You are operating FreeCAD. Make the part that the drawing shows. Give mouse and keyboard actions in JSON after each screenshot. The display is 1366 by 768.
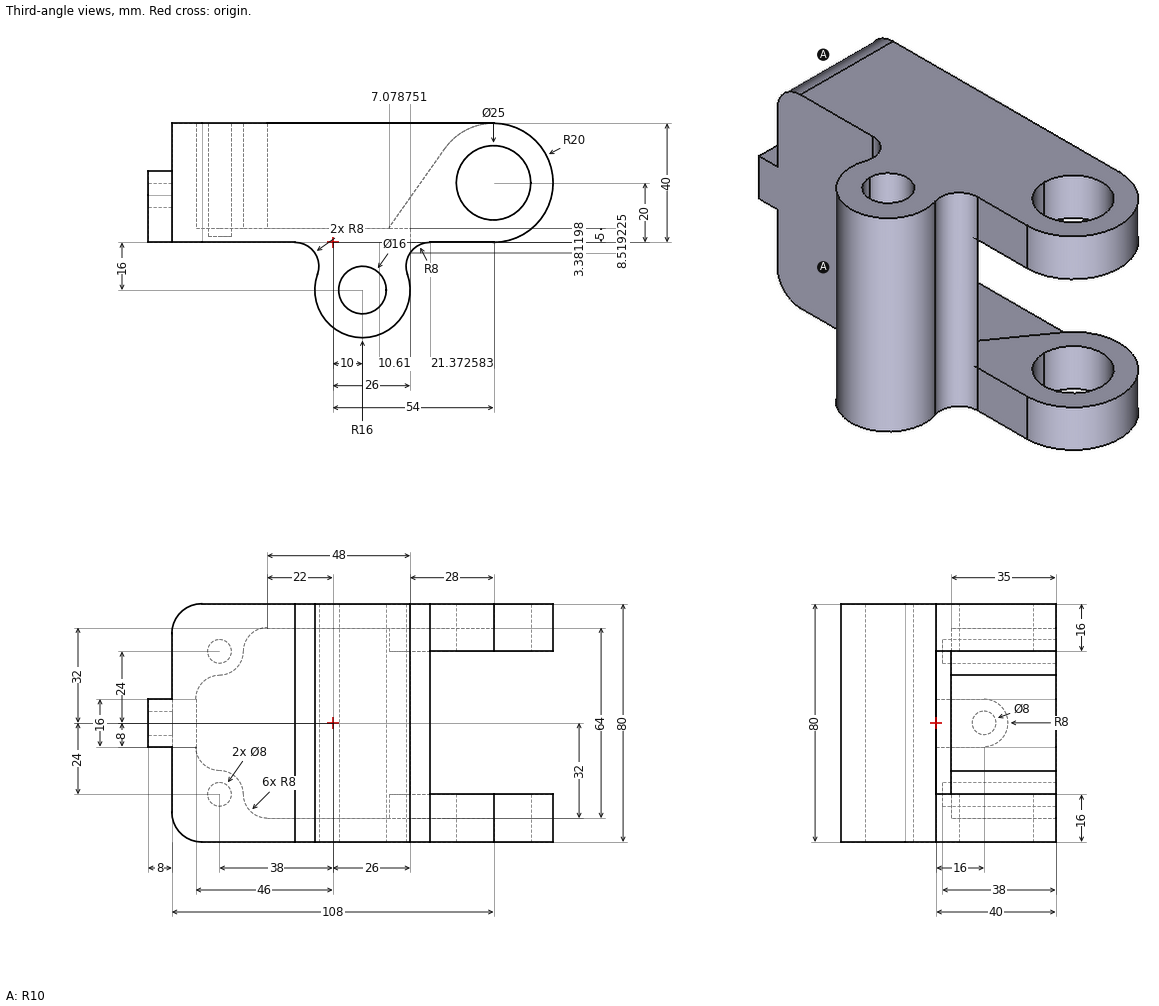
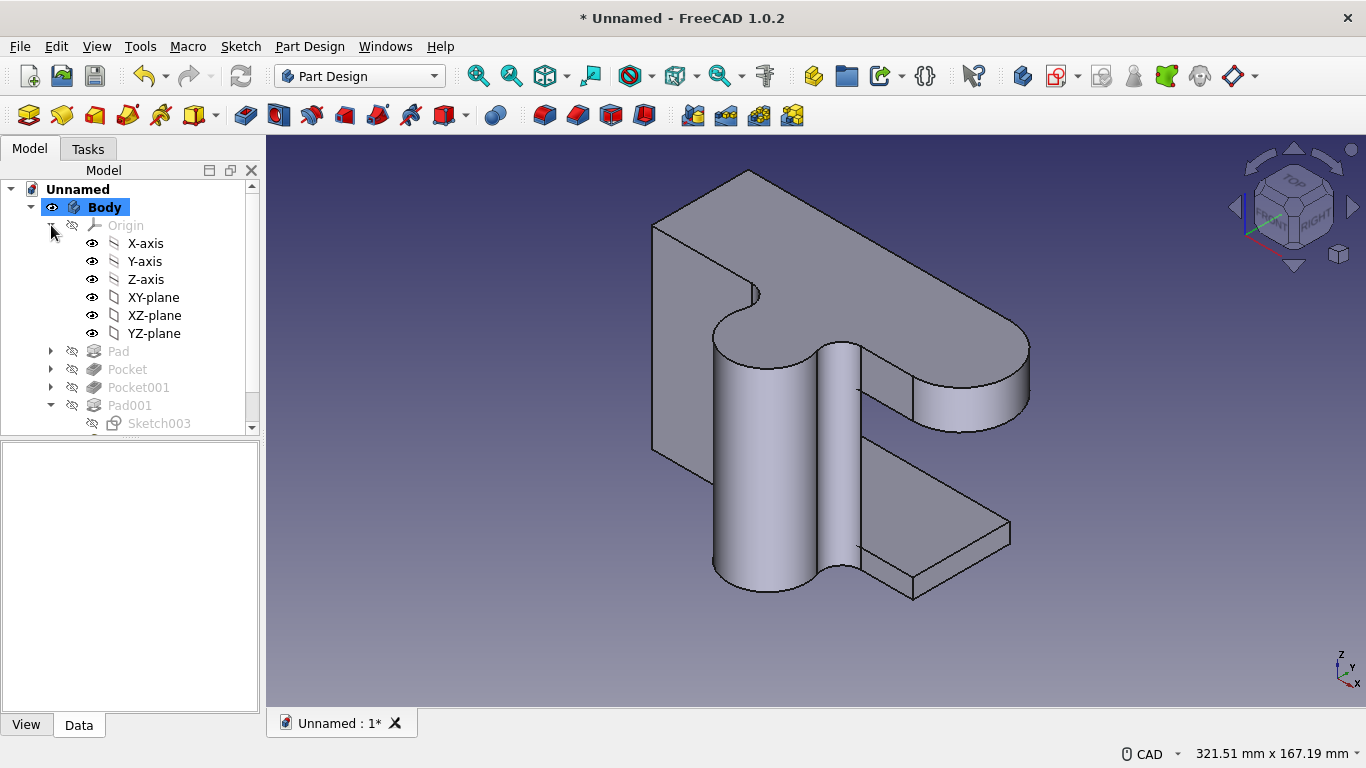
{"action": "left_click", "coordinate": [137, 297]}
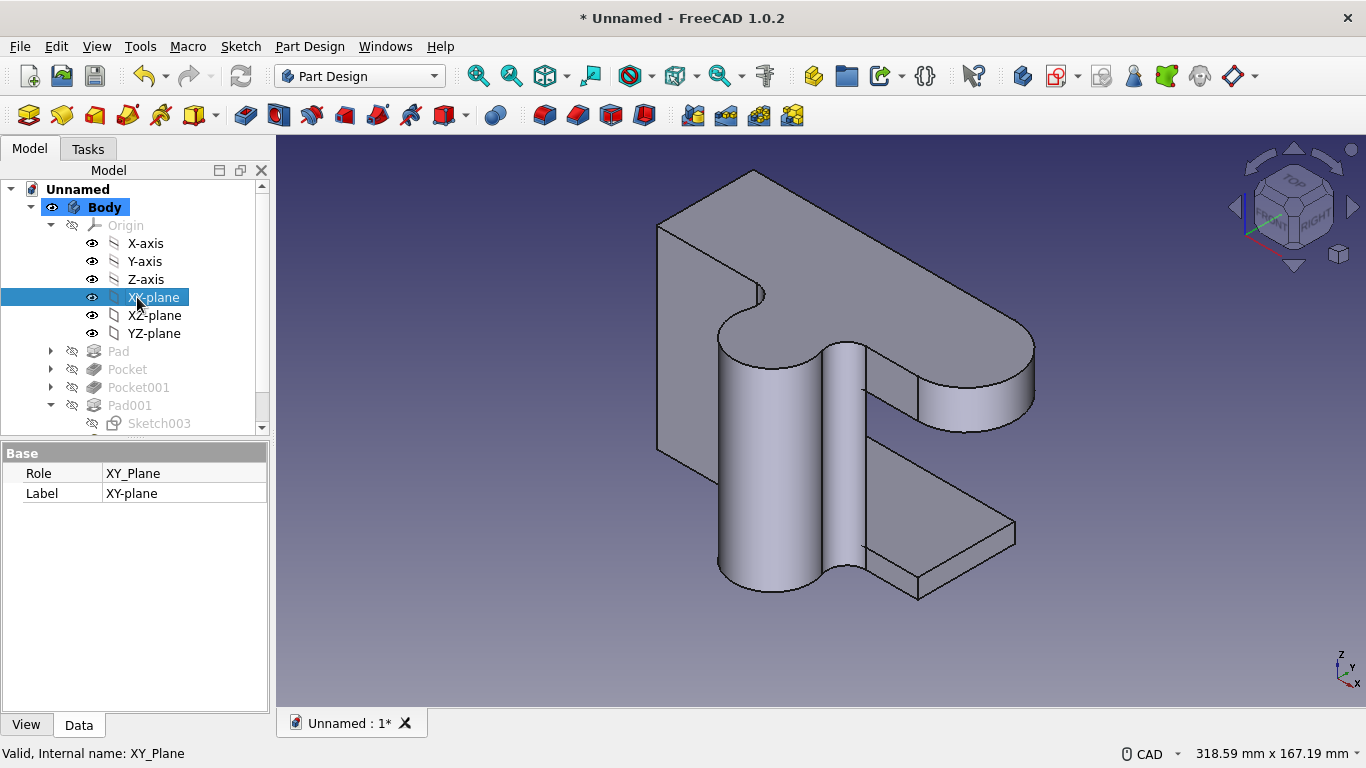
{"action": "left_click", "coordinate": [1232, 76]}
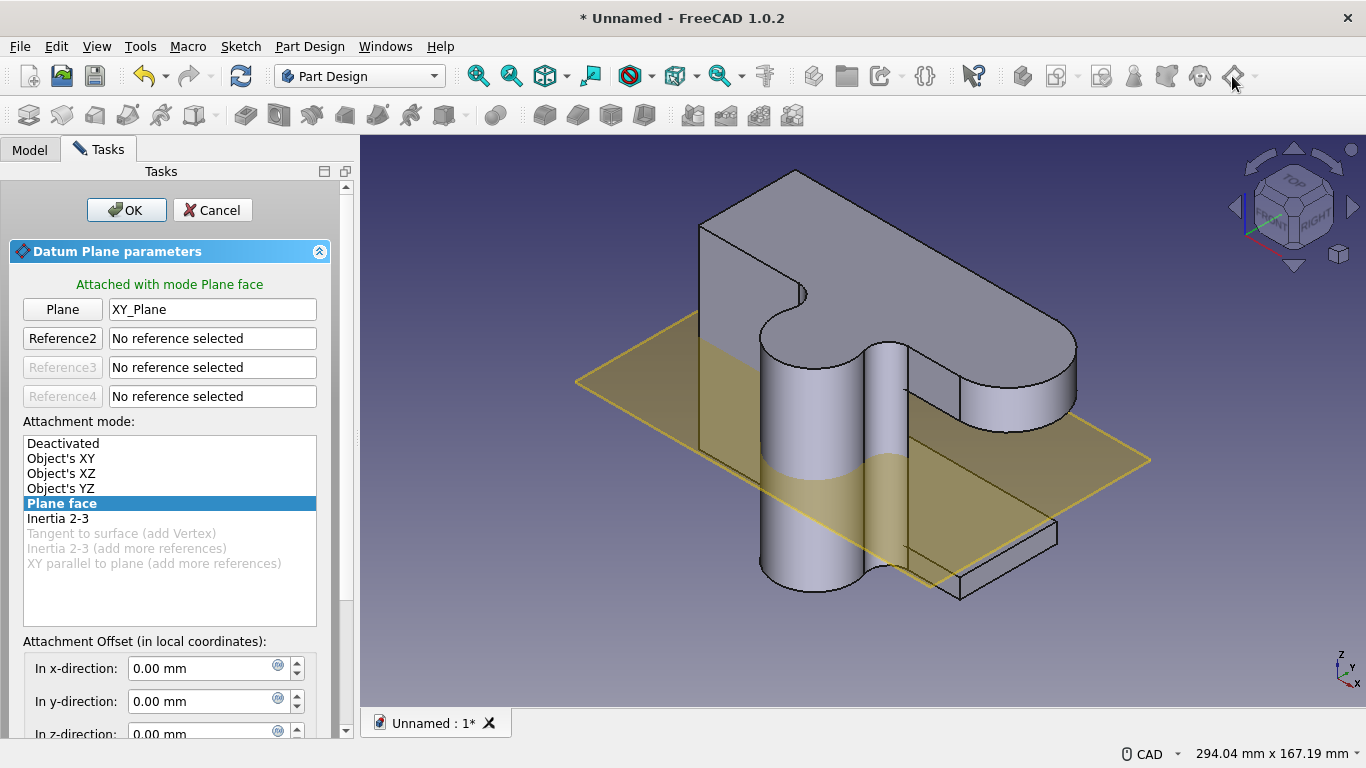
{"action": "scroll", "coordinate": [346, 460], "scroll_direction": "down", "scroll_amount": 2}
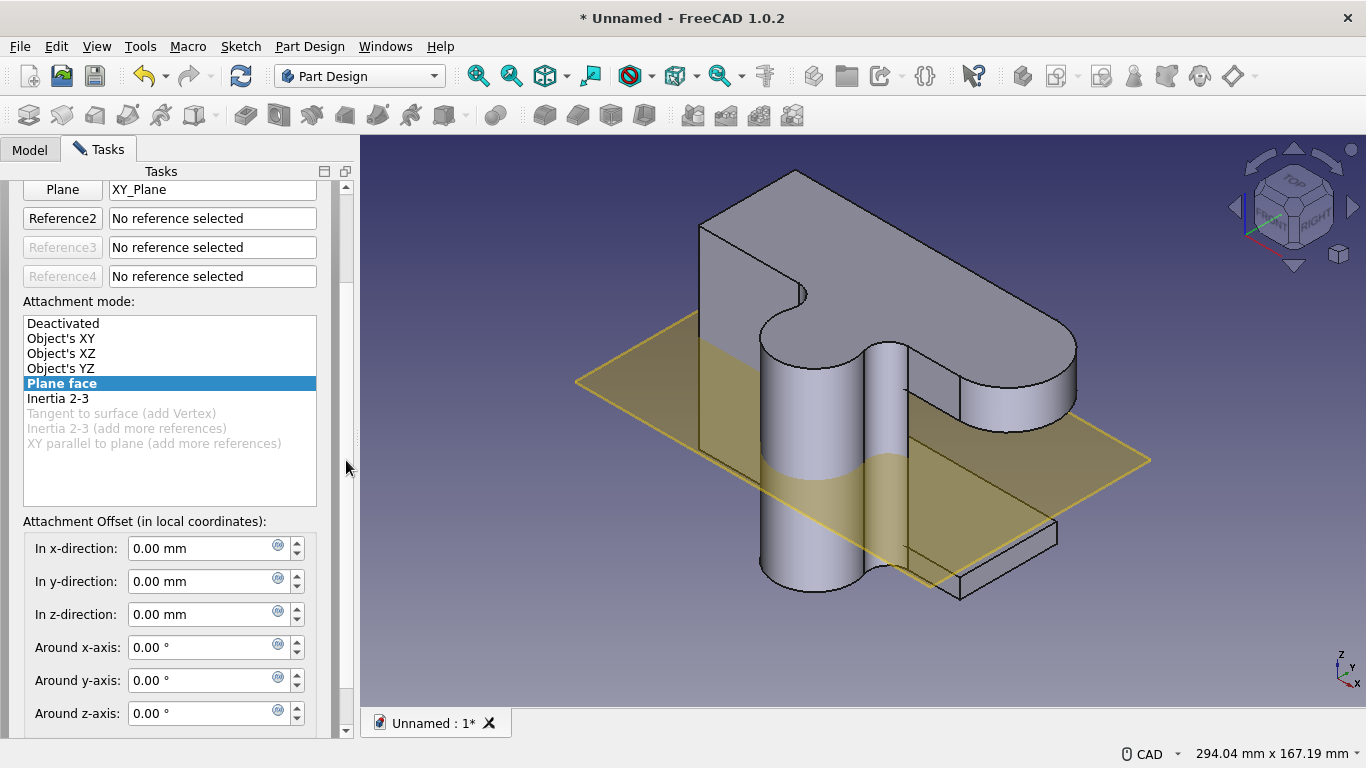
{"action": "triple_click", "coordinate": [210, 614]}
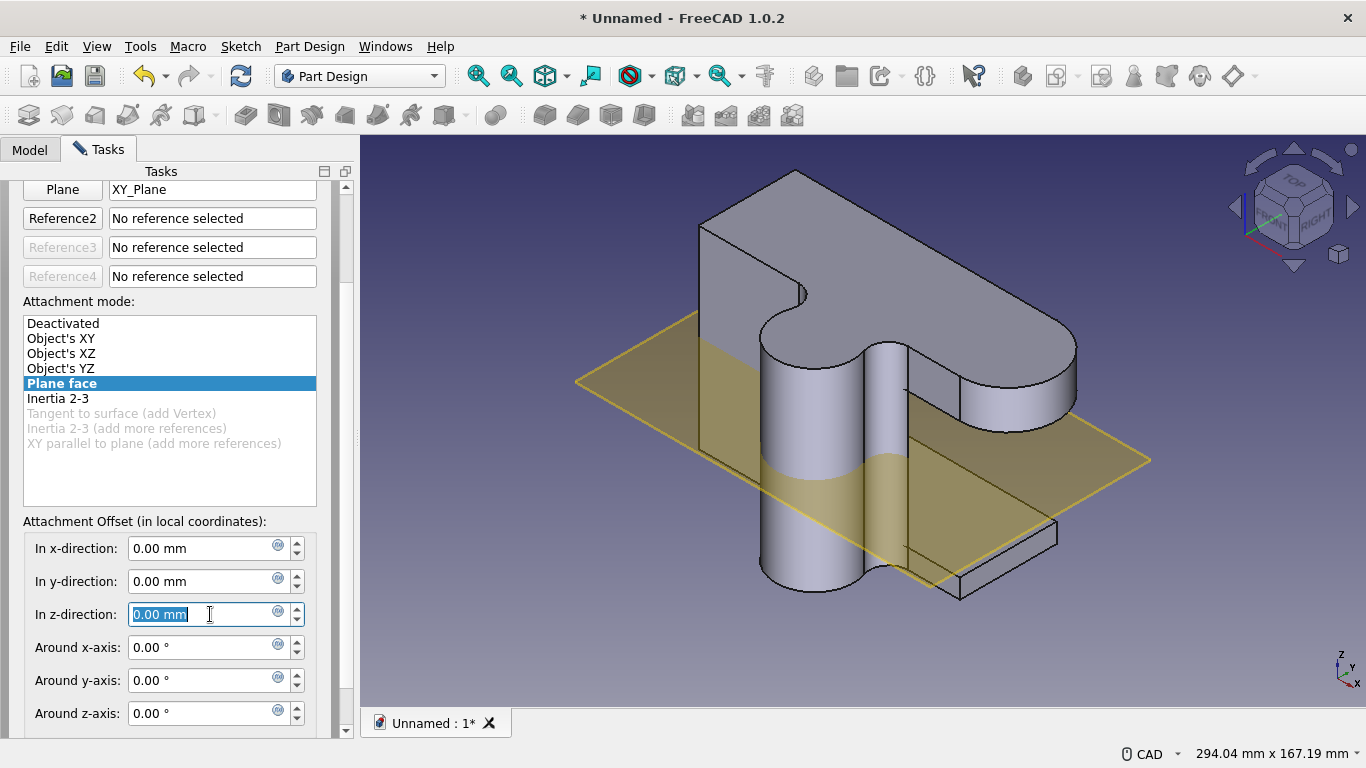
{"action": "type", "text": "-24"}
{"action": "key", "text": "Tab"}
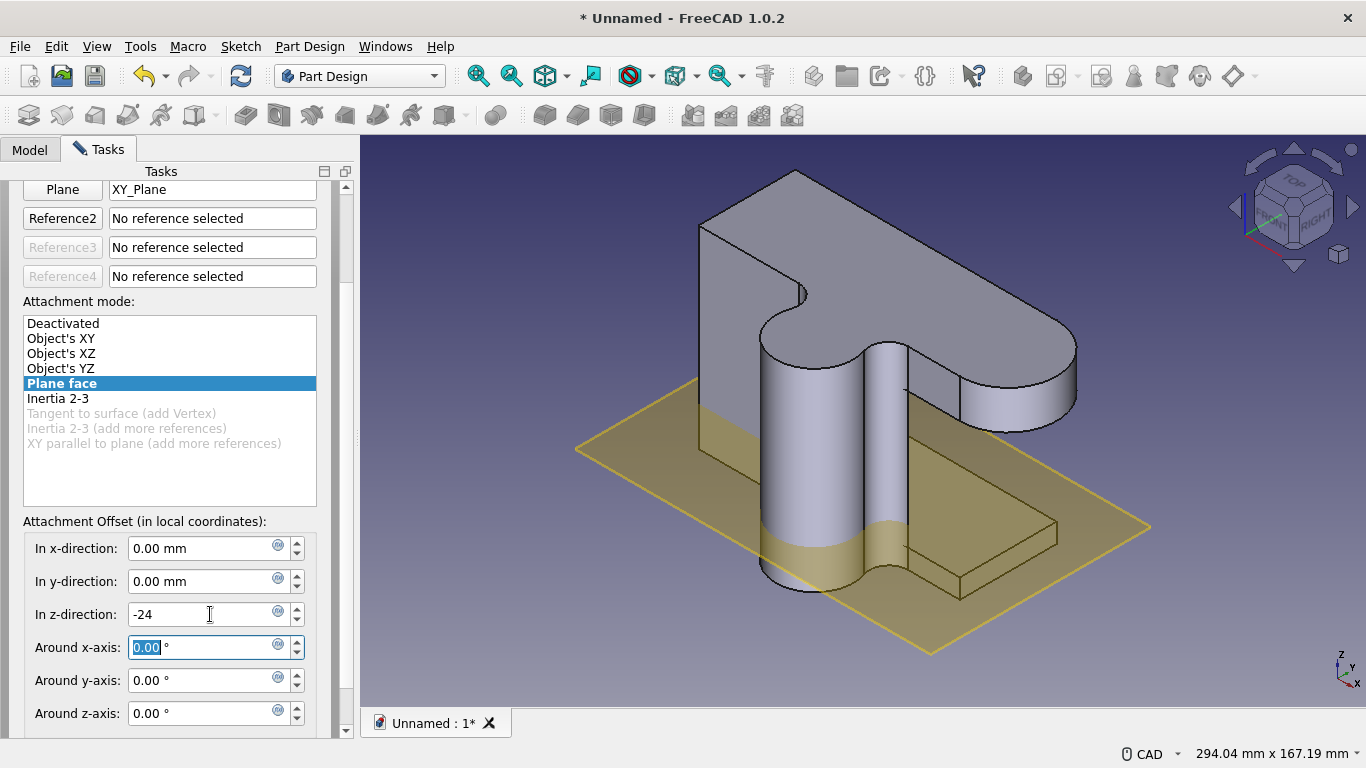
{"action": "scroll", "coordinate": [346, 460], "scroll_direction": "up", "scroll_amount": 3}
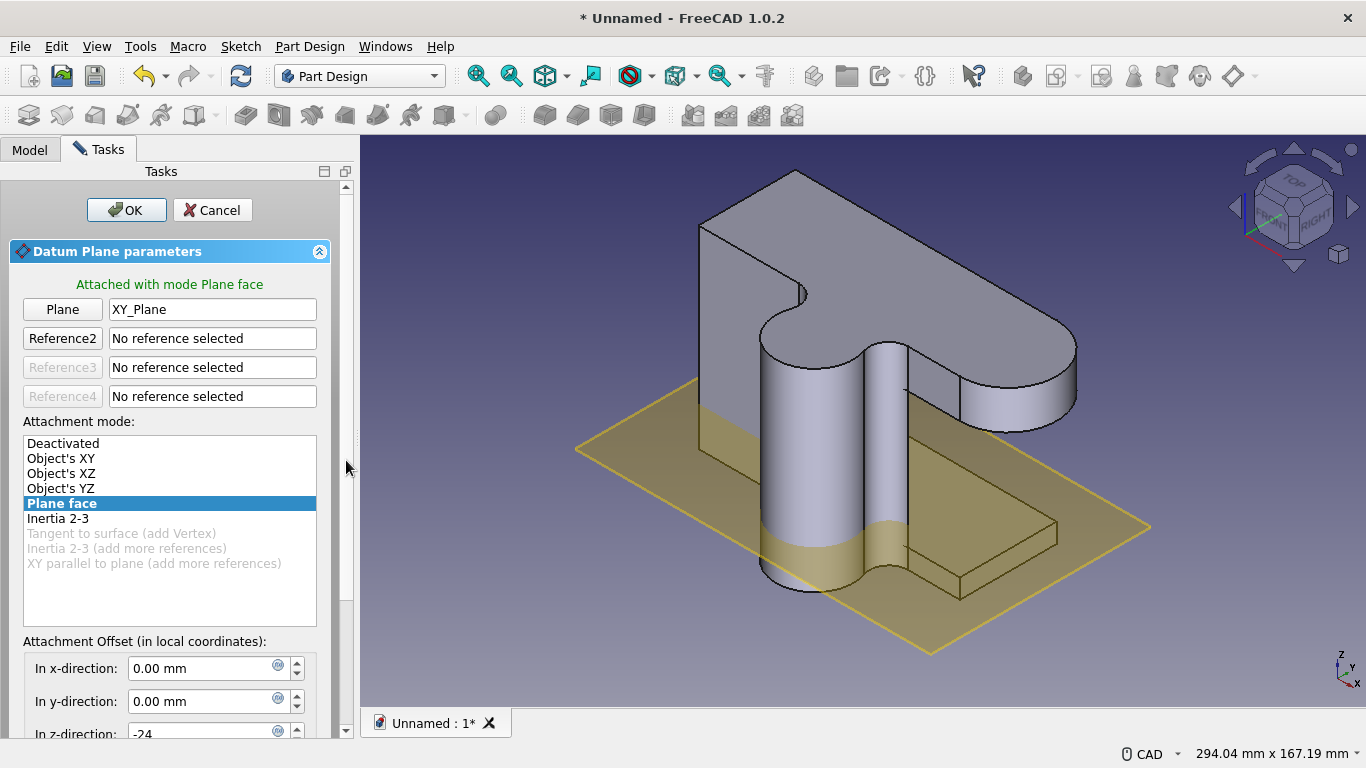
{"action": "left_click", "coordinate": [127, 210]}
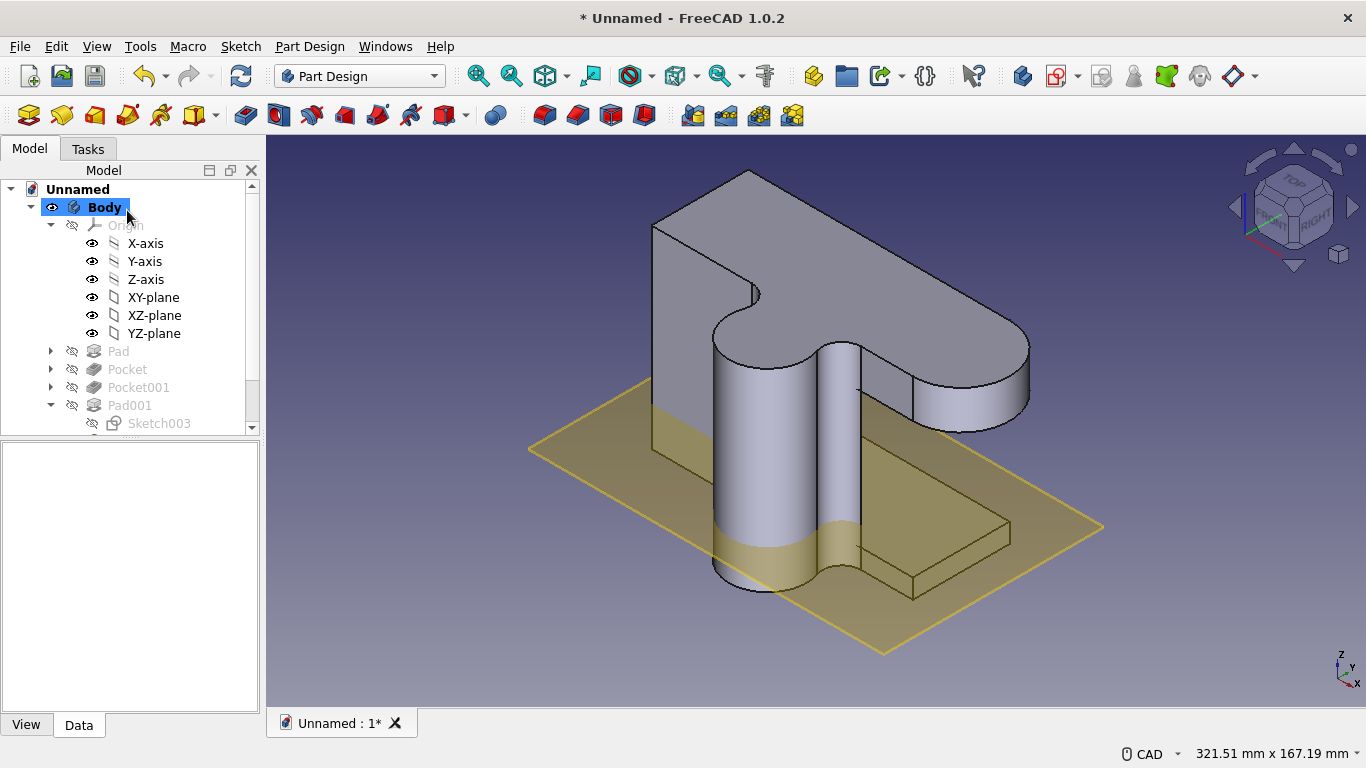
{"action": "scroll", "coordinate": [101, 311], "scroll_direction": "down", "scroll_amount": 3}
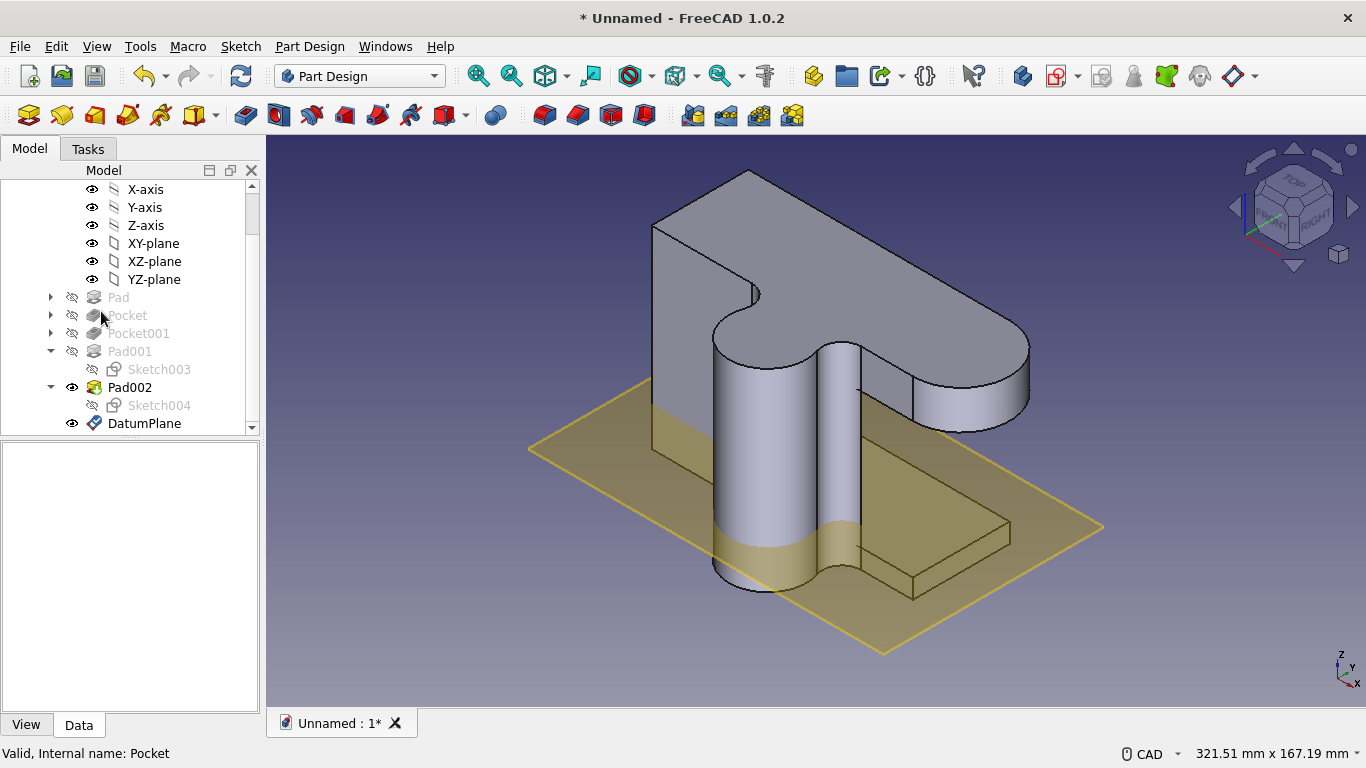
{"action": "left_click", "coordinate": [117, 423]}